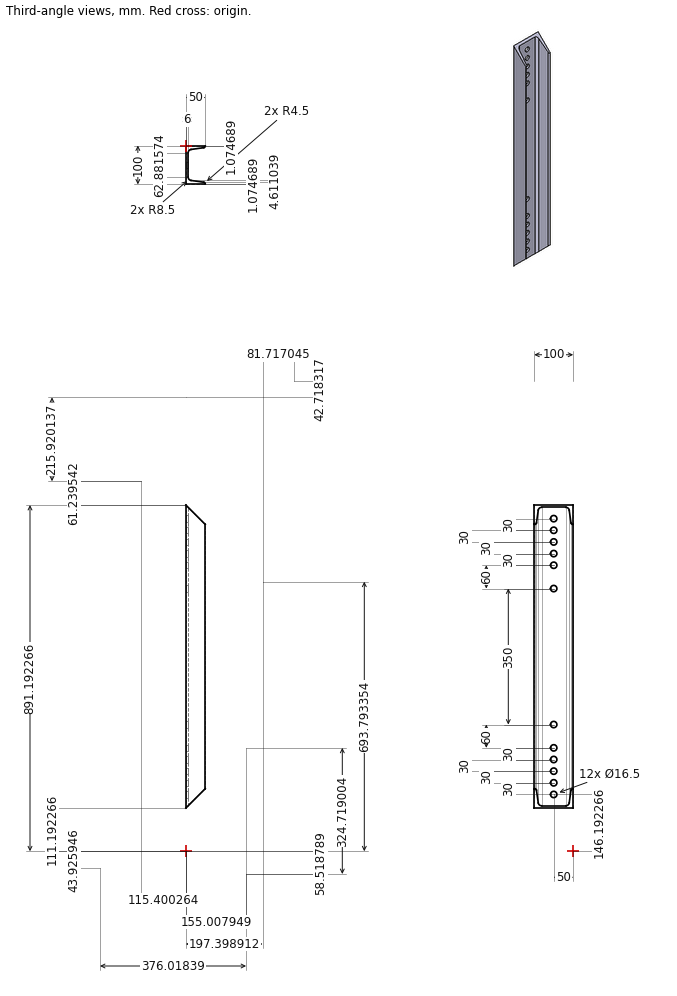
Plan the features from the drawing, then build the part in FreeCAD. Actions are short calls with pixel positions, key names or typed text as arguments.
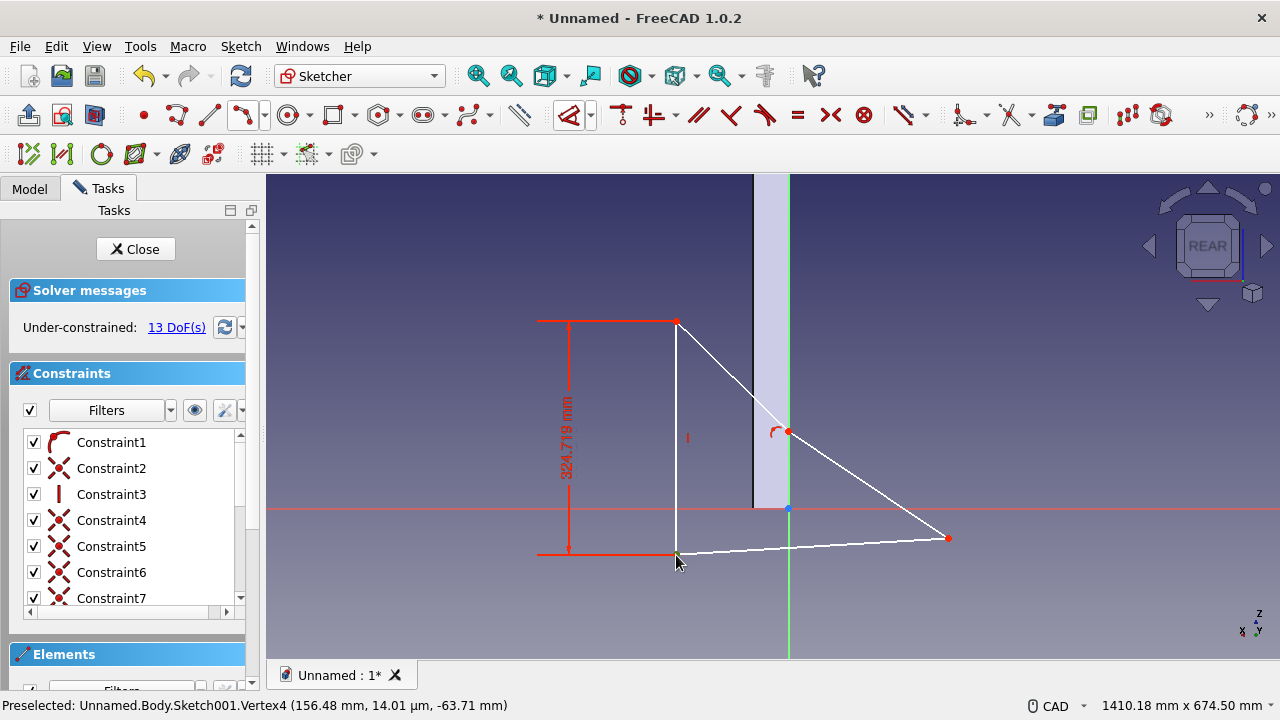
click(590, 116)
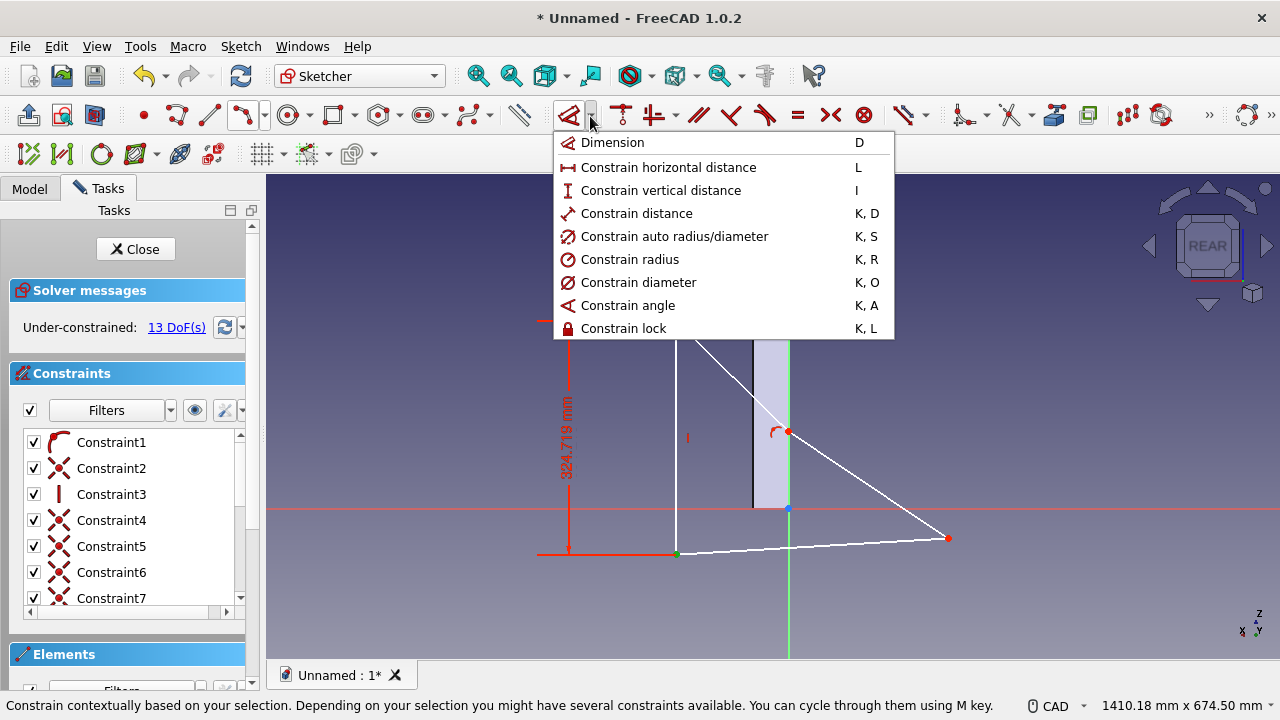
click(724, 190)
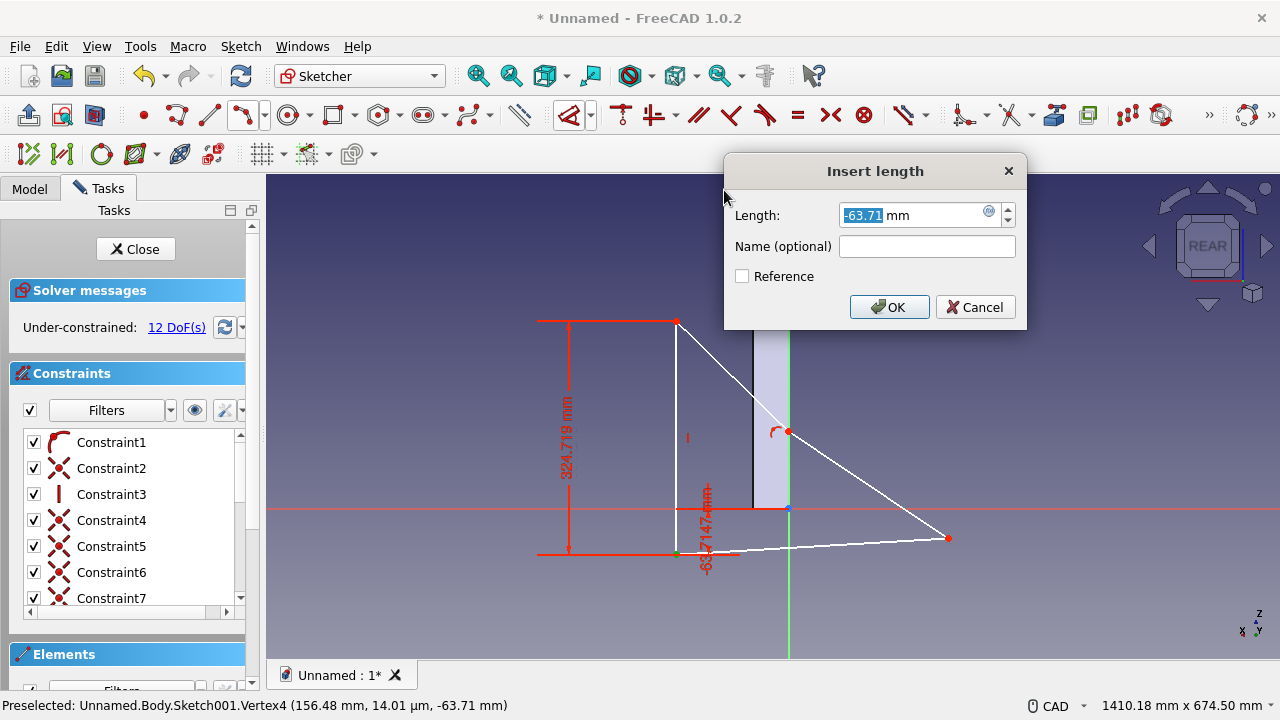
text(-58.518789)
key(Return)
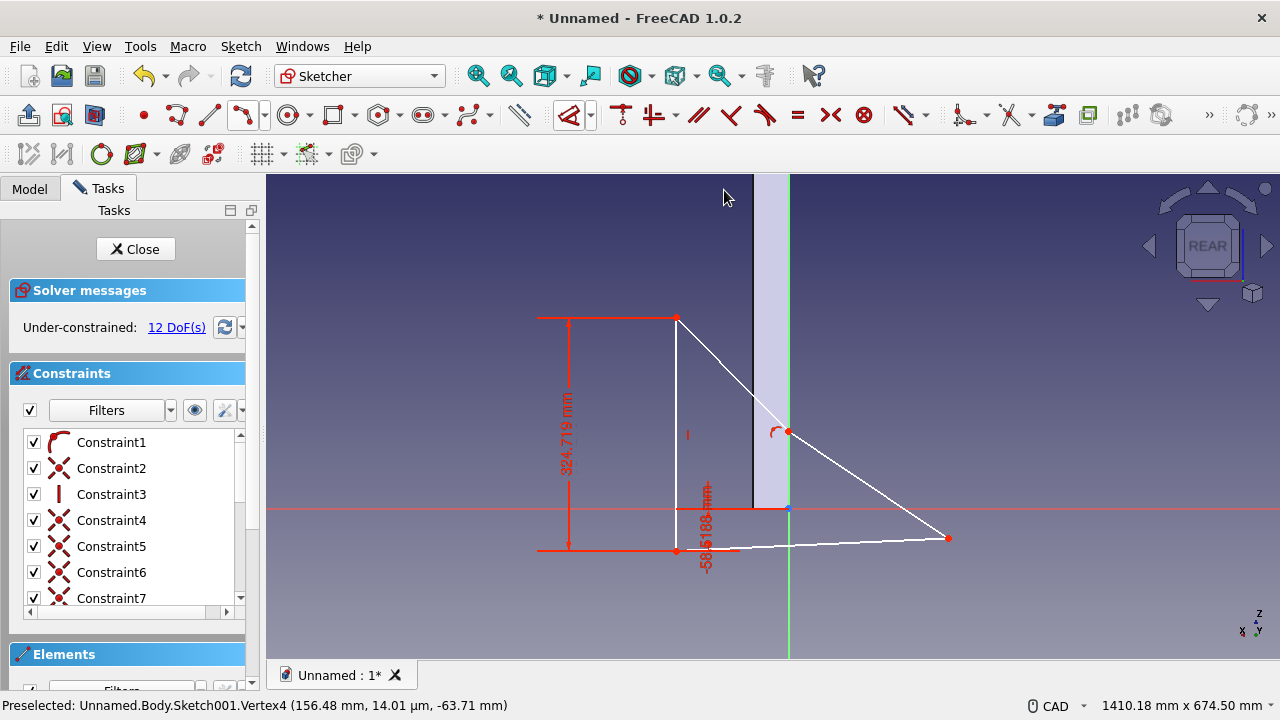
scroll(948, 538, up, 2)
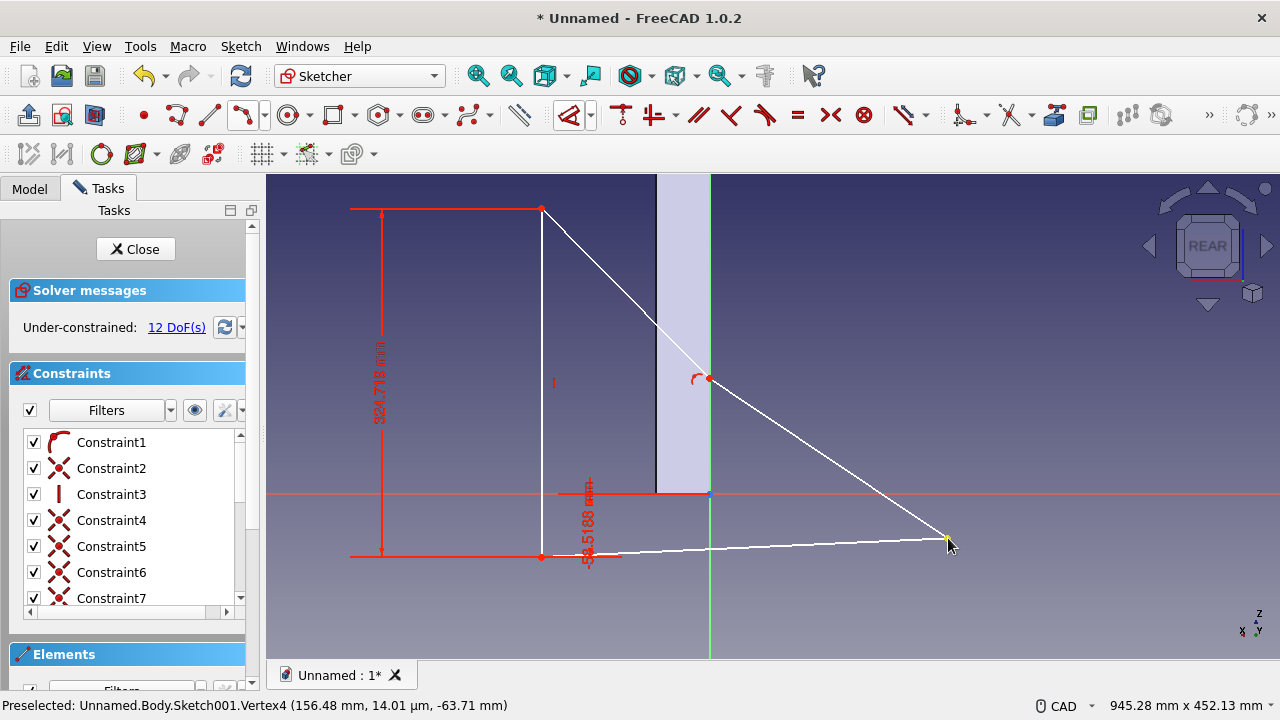
click(948, 538)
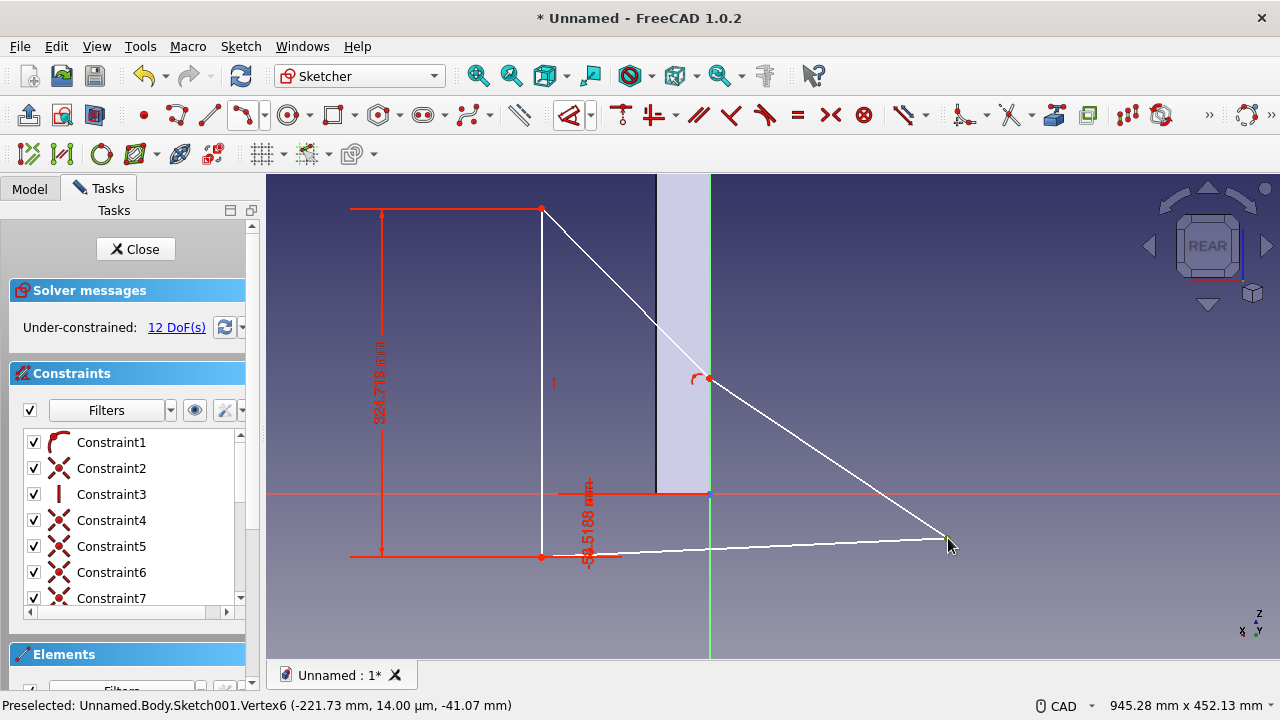
key(i)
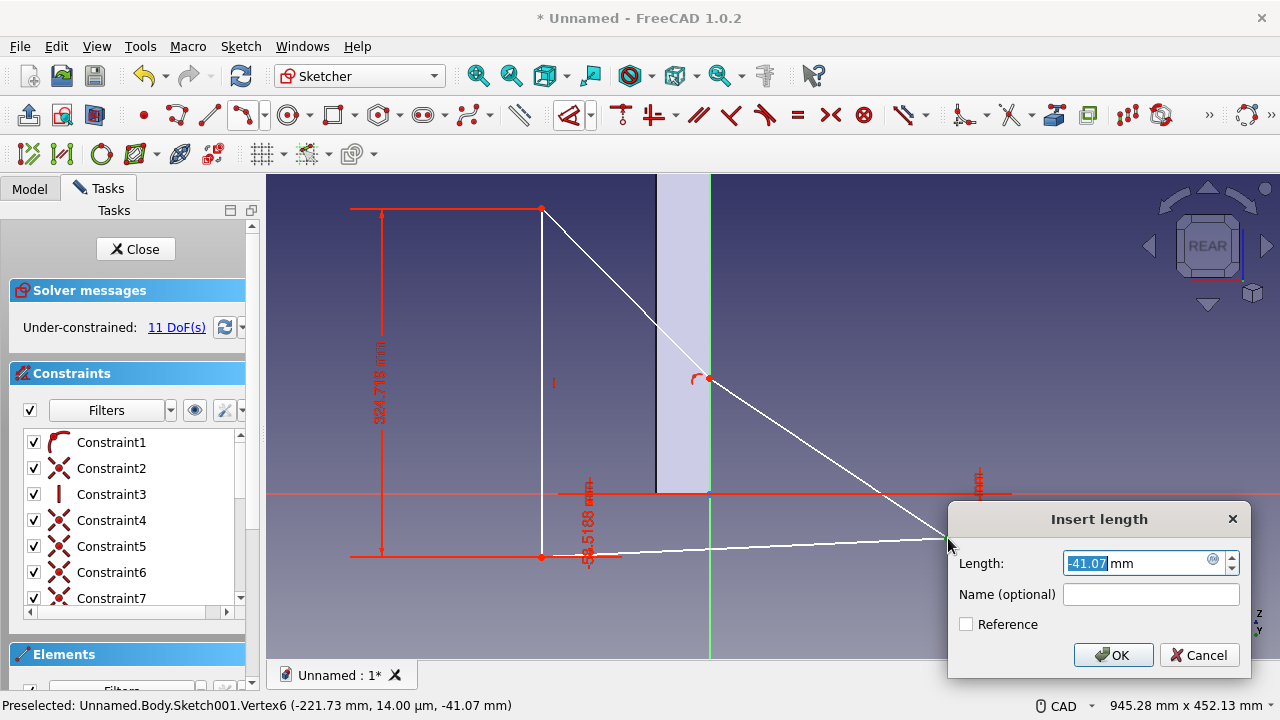
text(-43.925946)
key(Return)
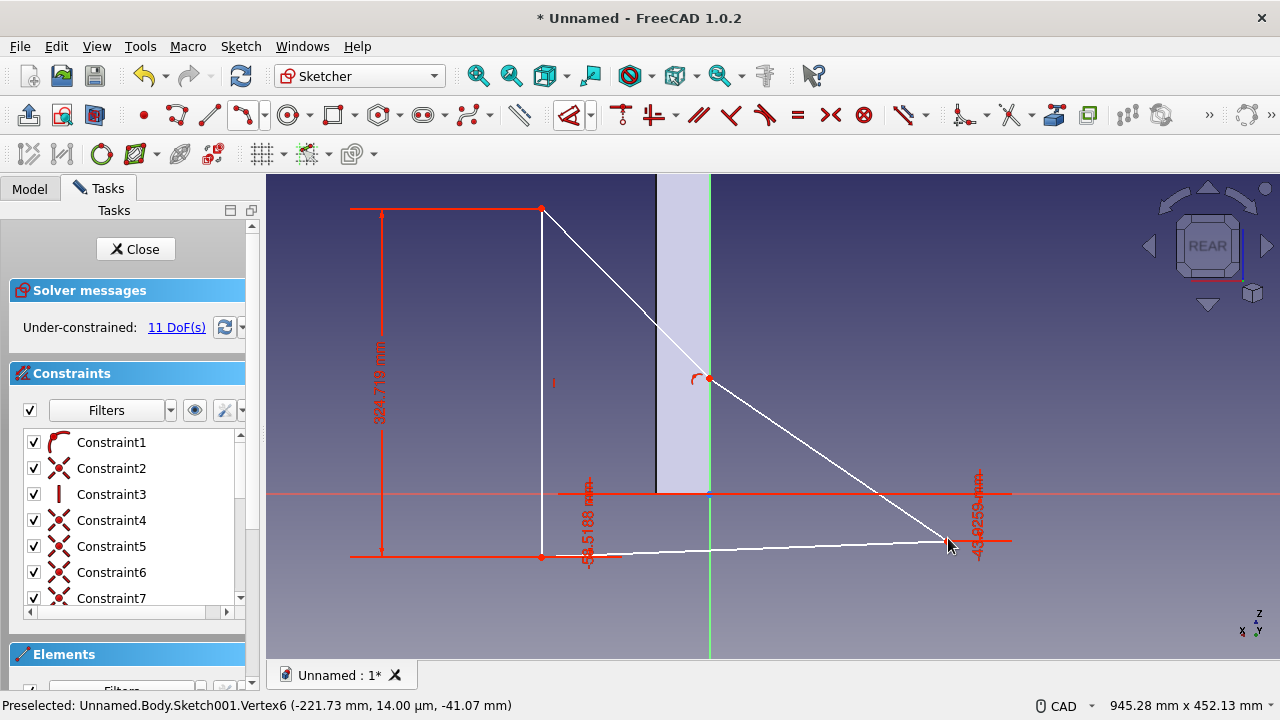
scroll(711, 553, down, 8)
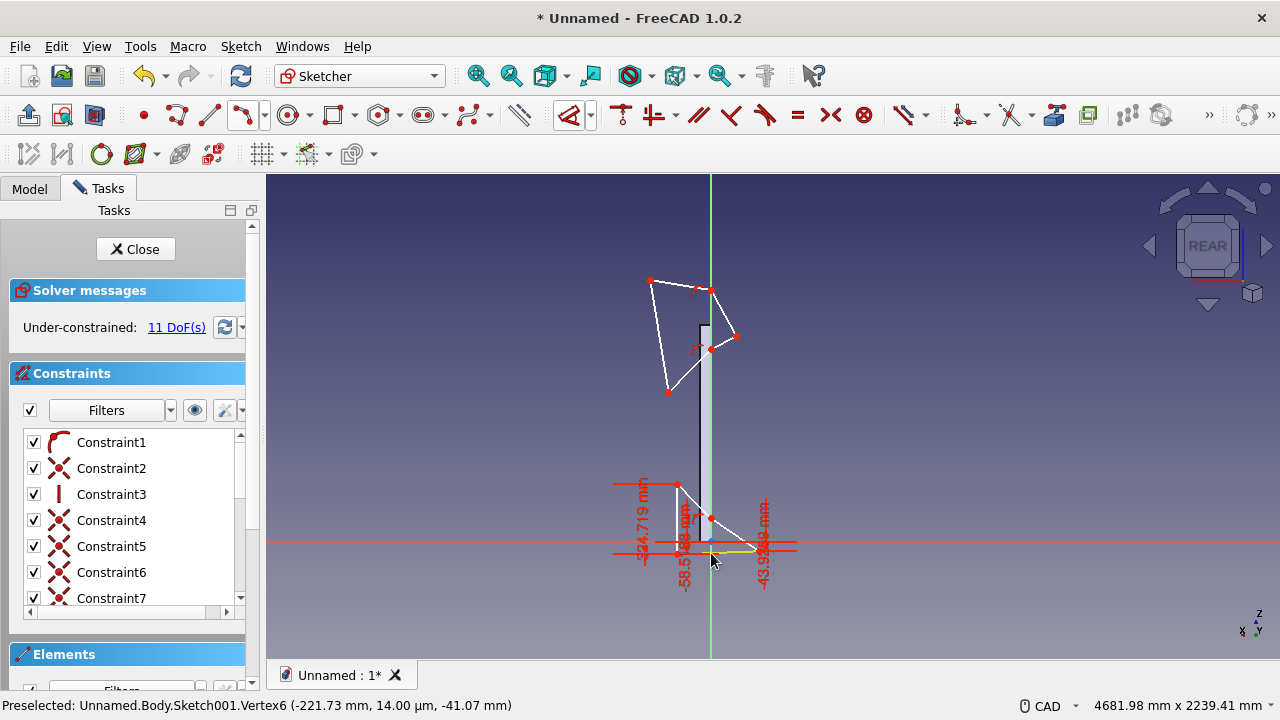
scroll(702, 553, up, 2)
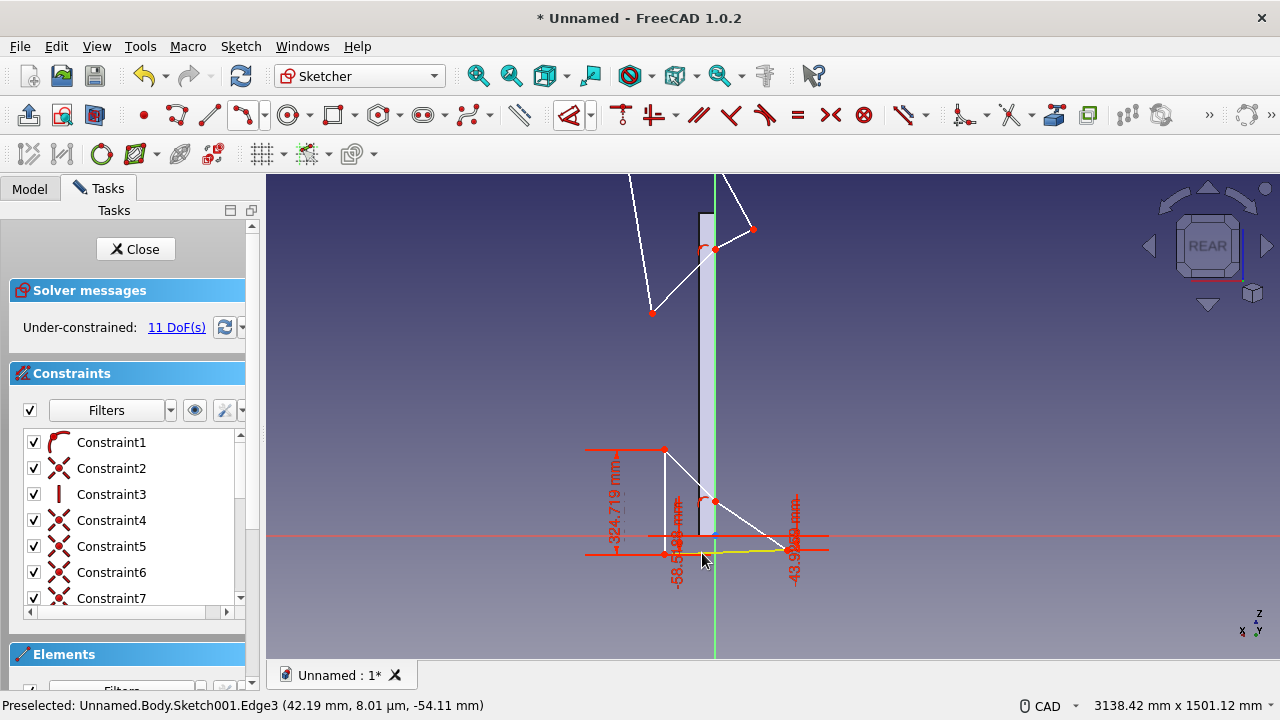
click(701, 553)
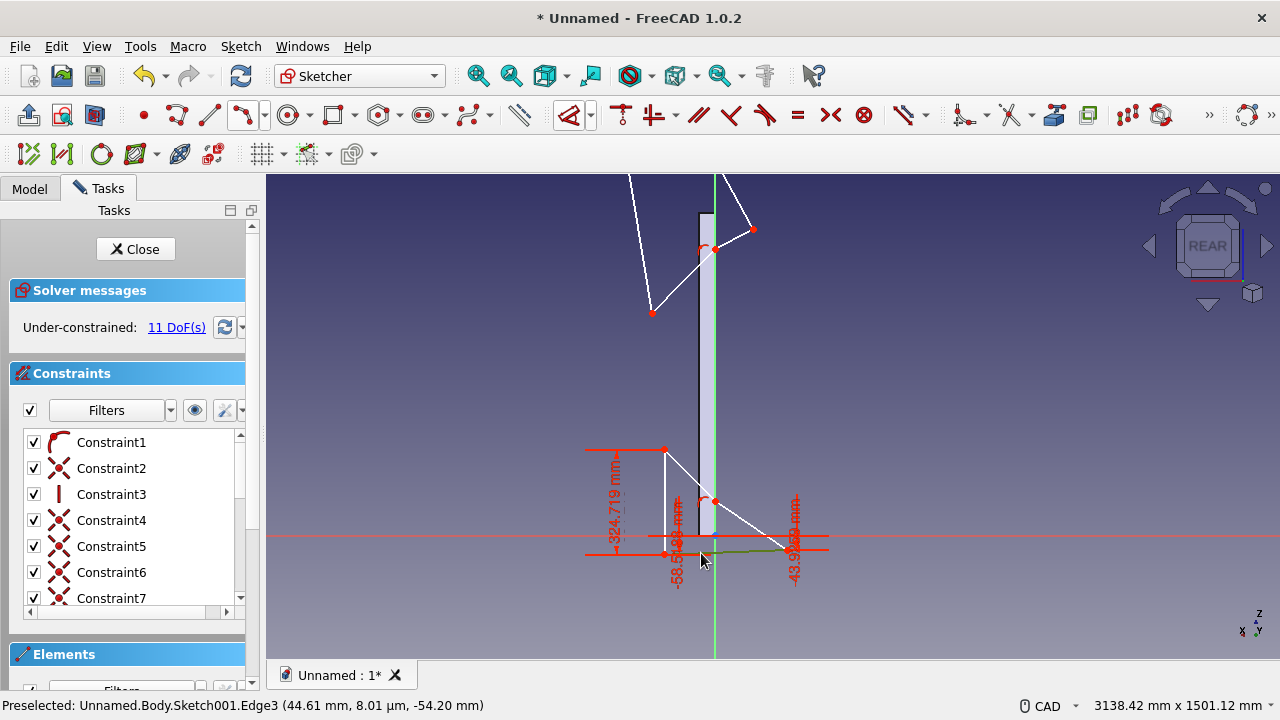
click(590, 116)